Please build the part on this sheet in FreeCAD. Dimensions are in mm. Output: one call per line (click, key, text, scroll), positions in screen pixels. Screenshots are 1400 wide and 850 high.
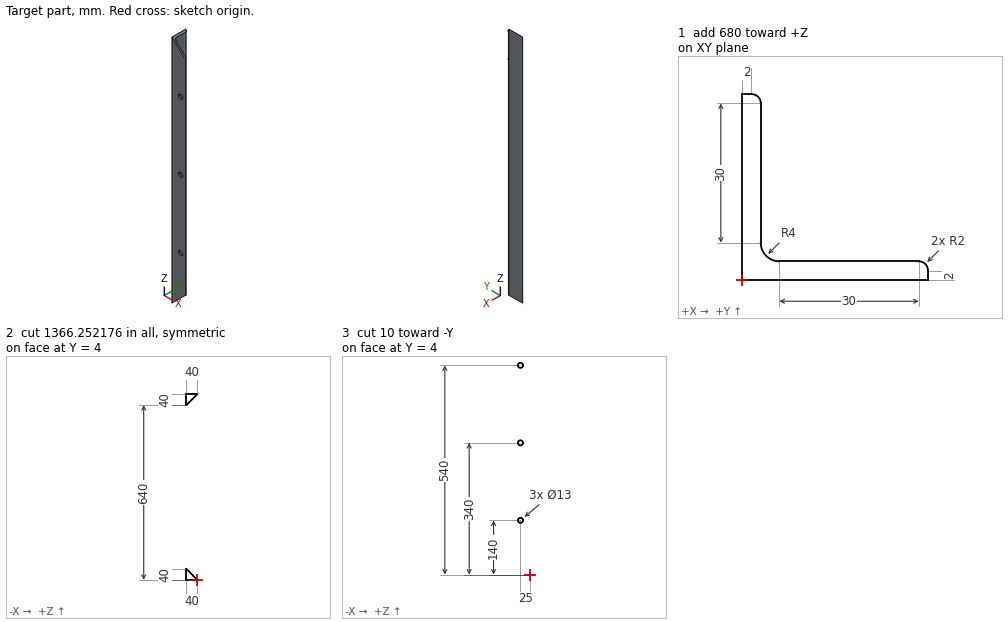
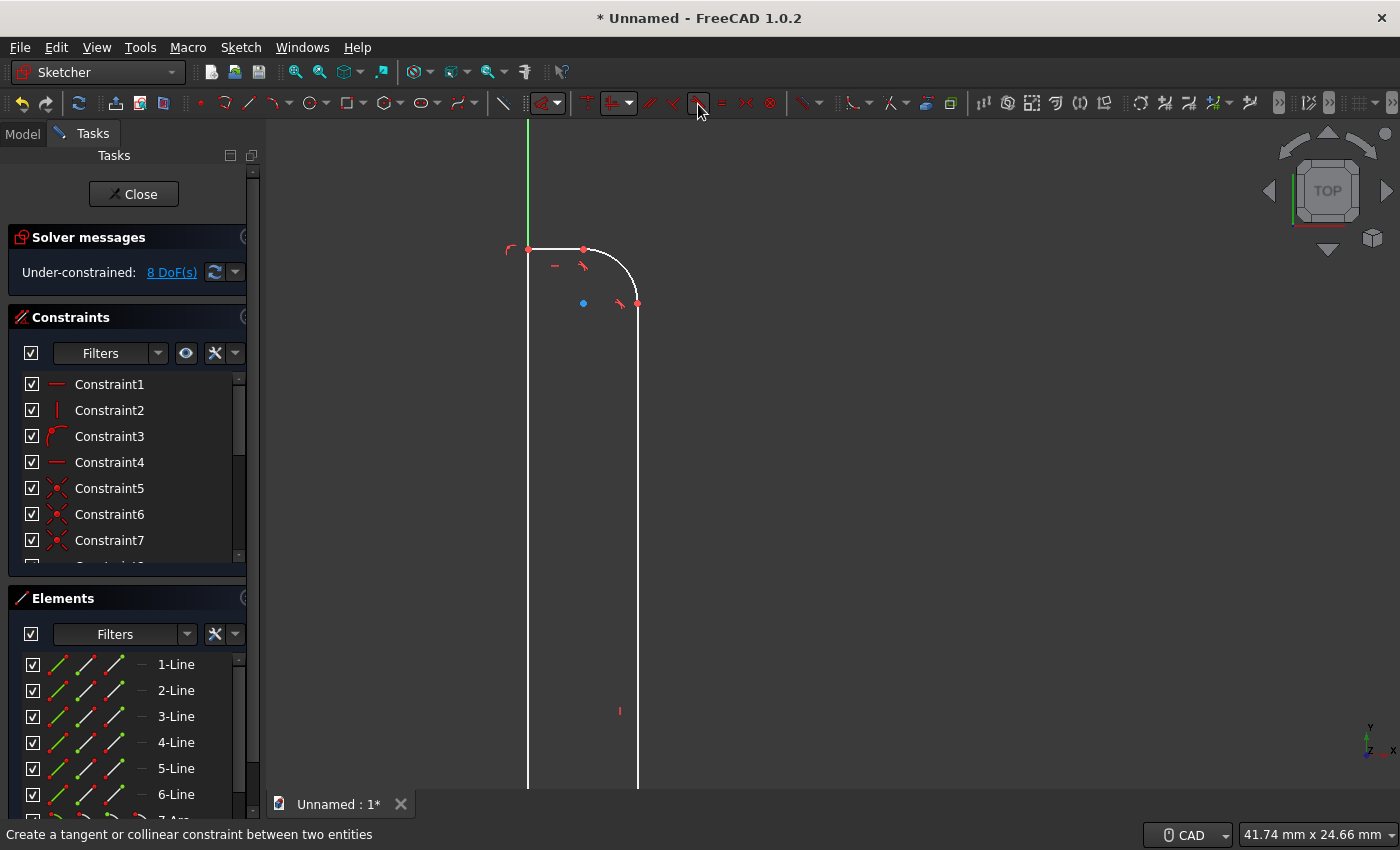
scroll(586, 258, down, 5)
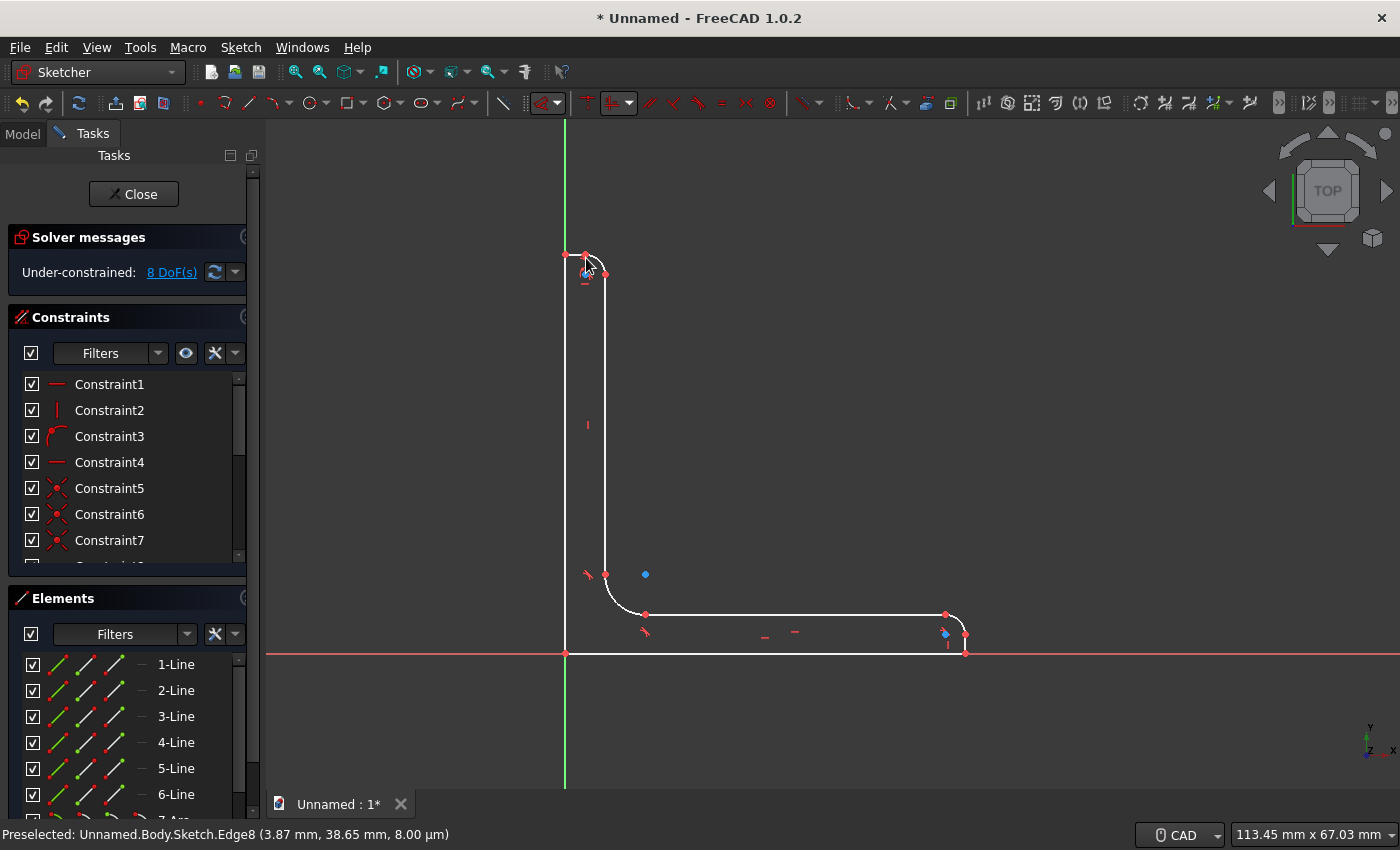
scroll(965, 648, up, 5)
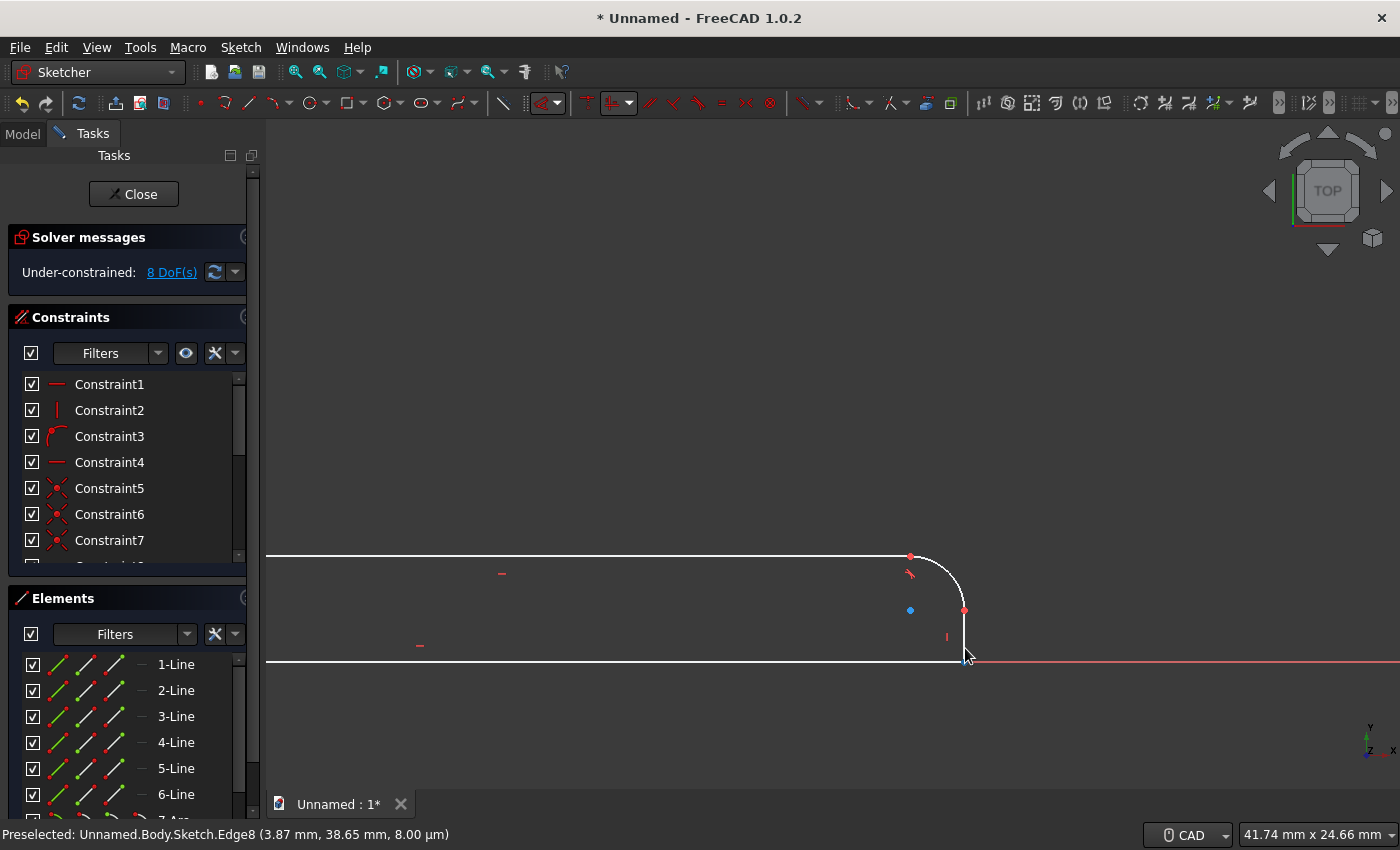
click(964, 647)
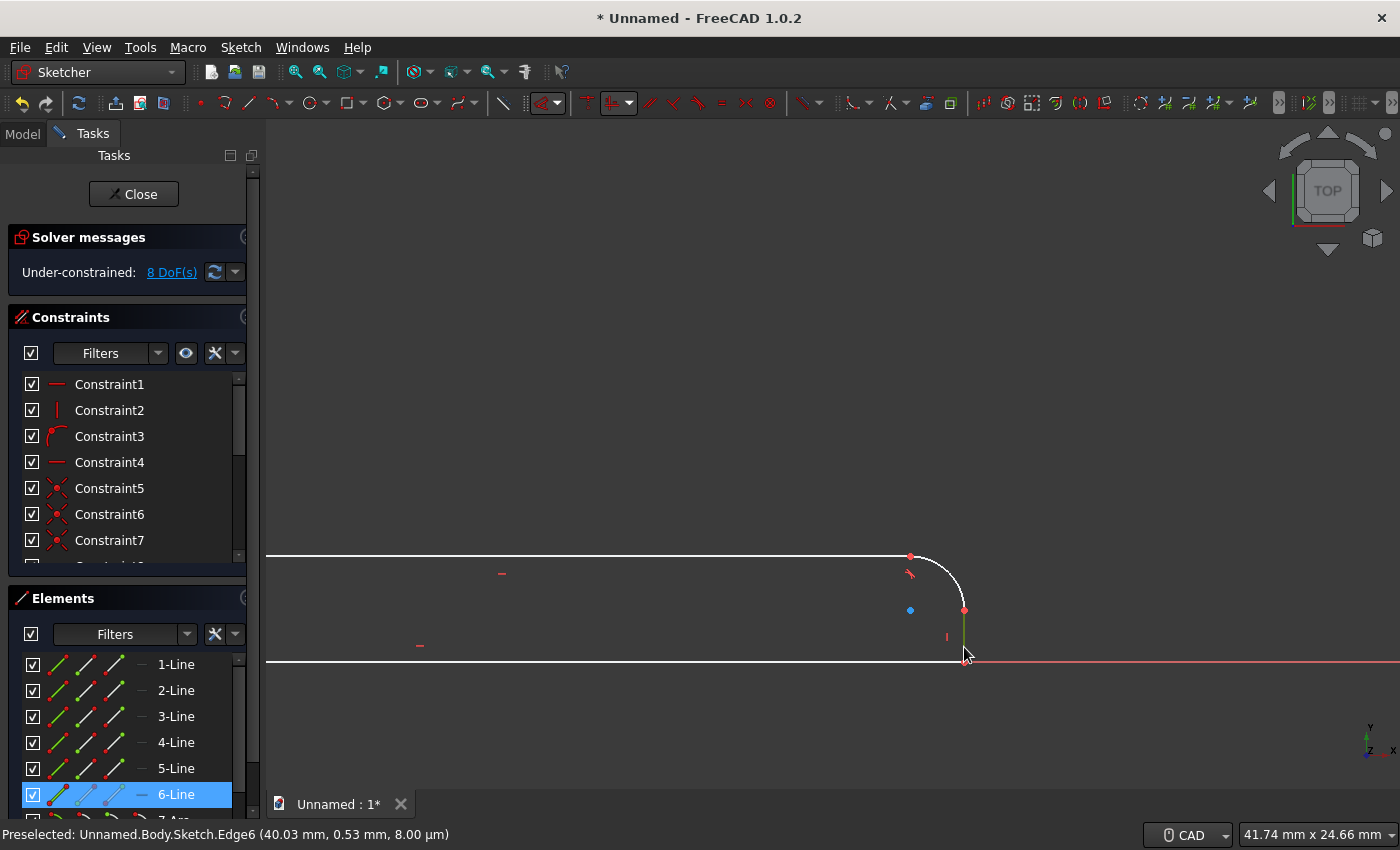
click(958, 586)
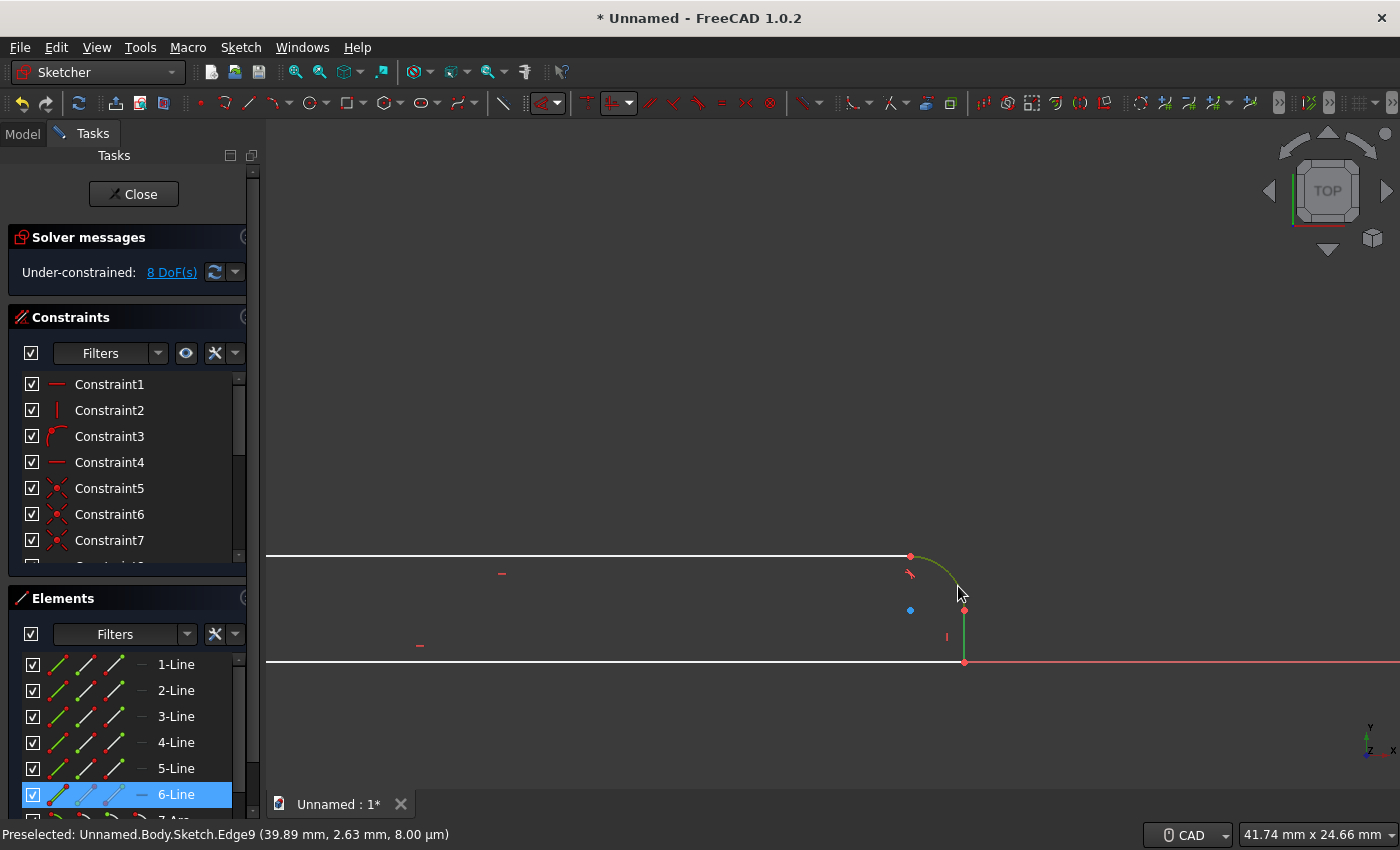
click(698, 104)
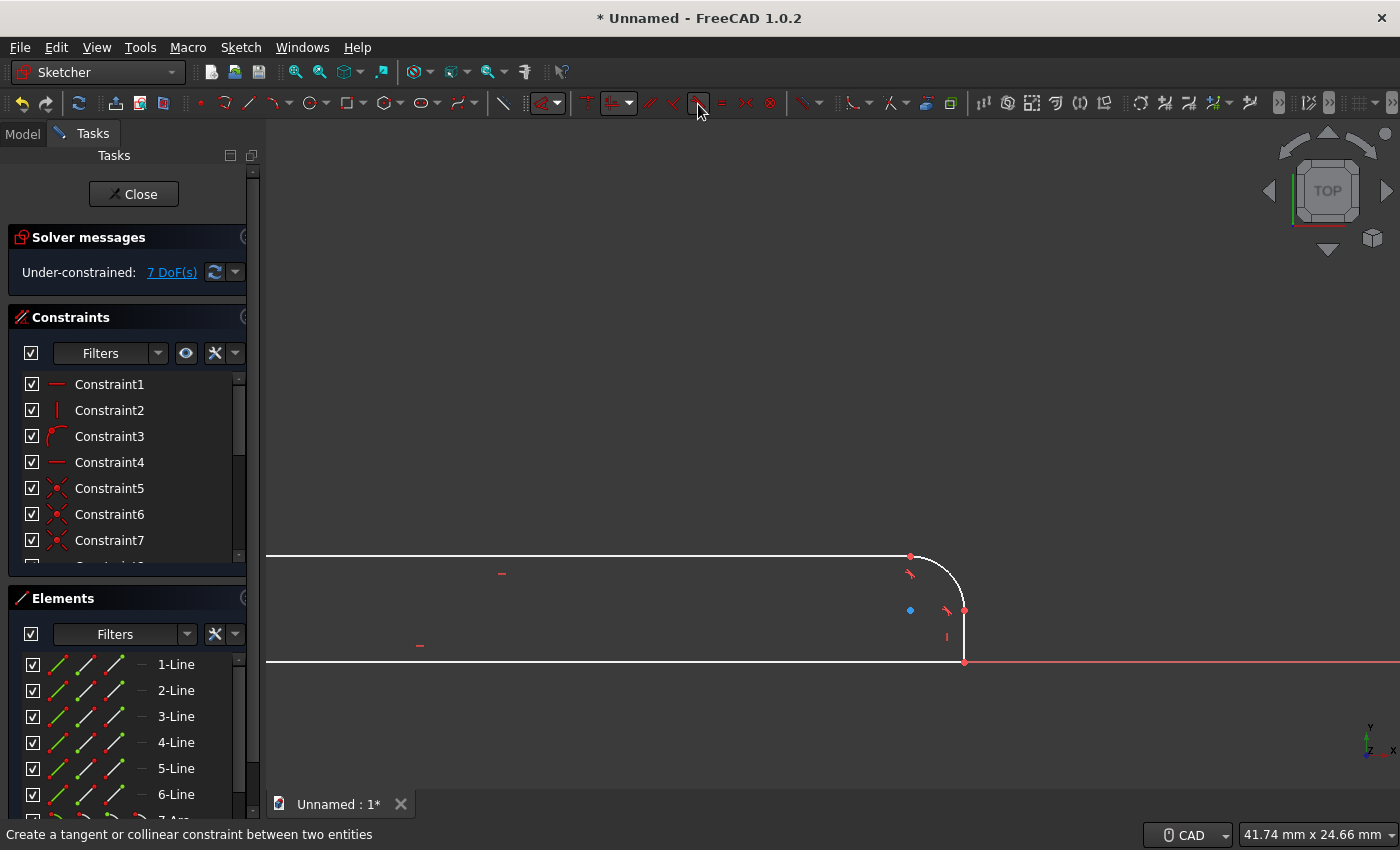
scroll(965, 649, down, 5)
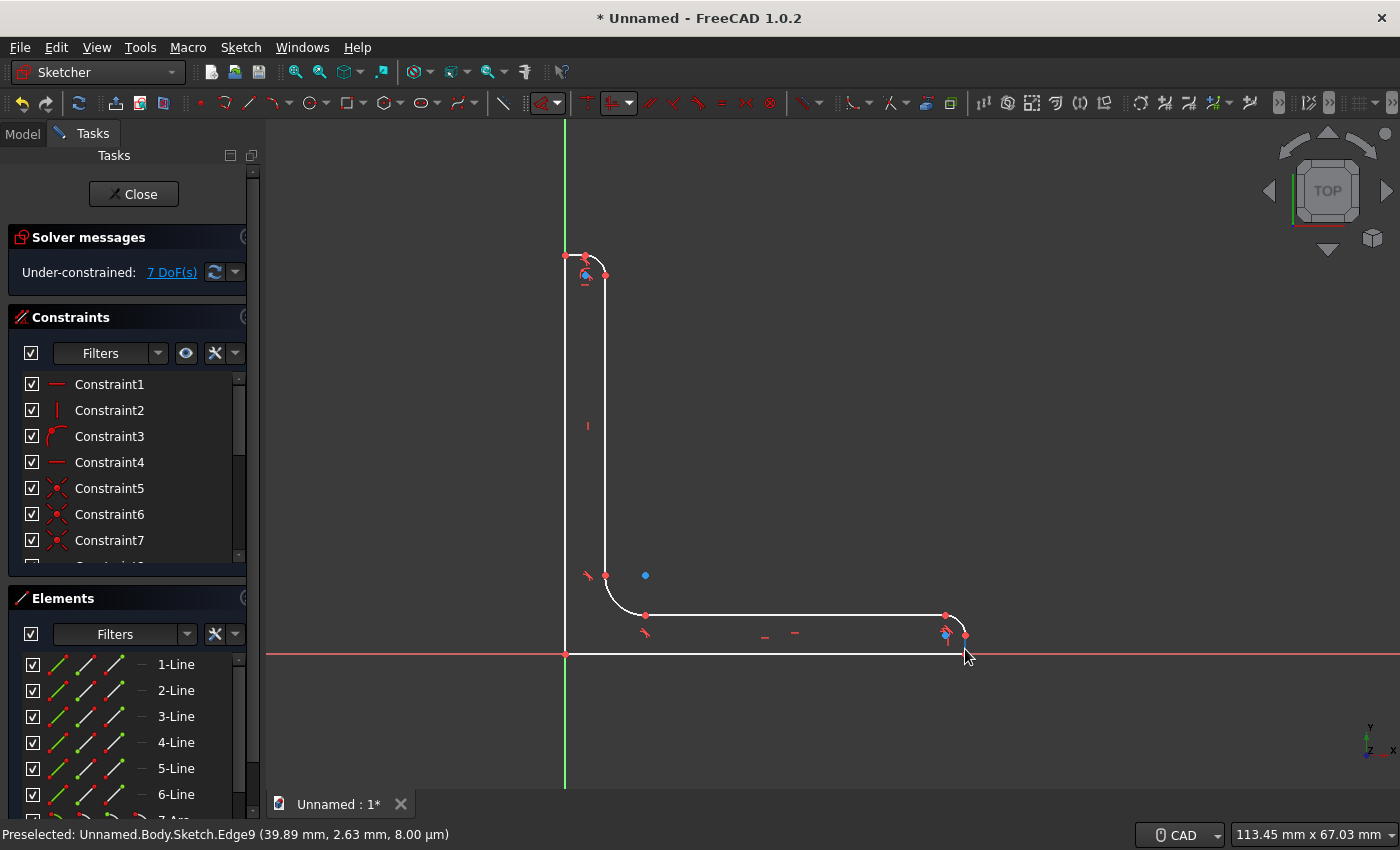
scroll(603, 266, up, 2)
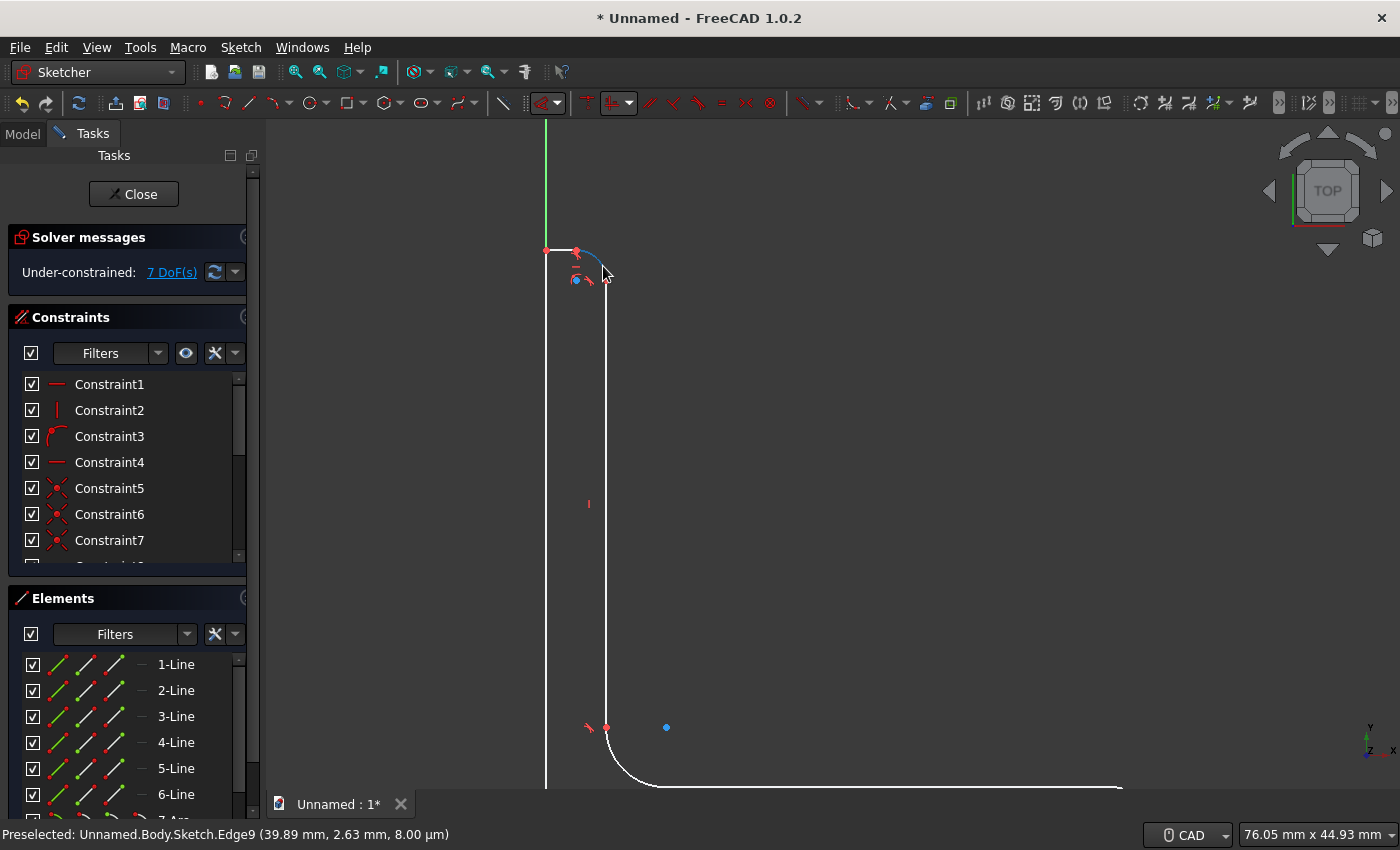
click(603, 266)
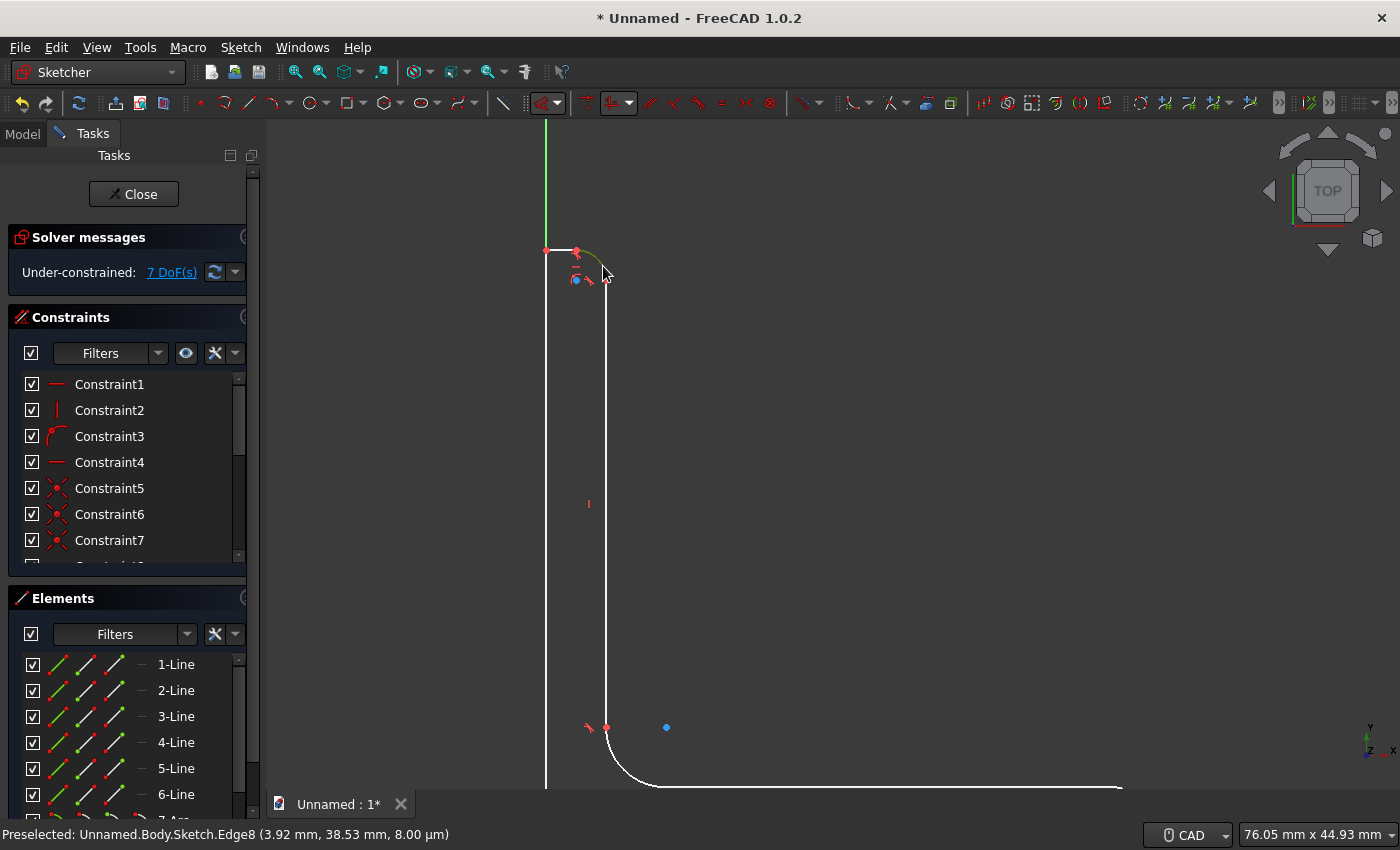
scroll(602, 265, down, 2)